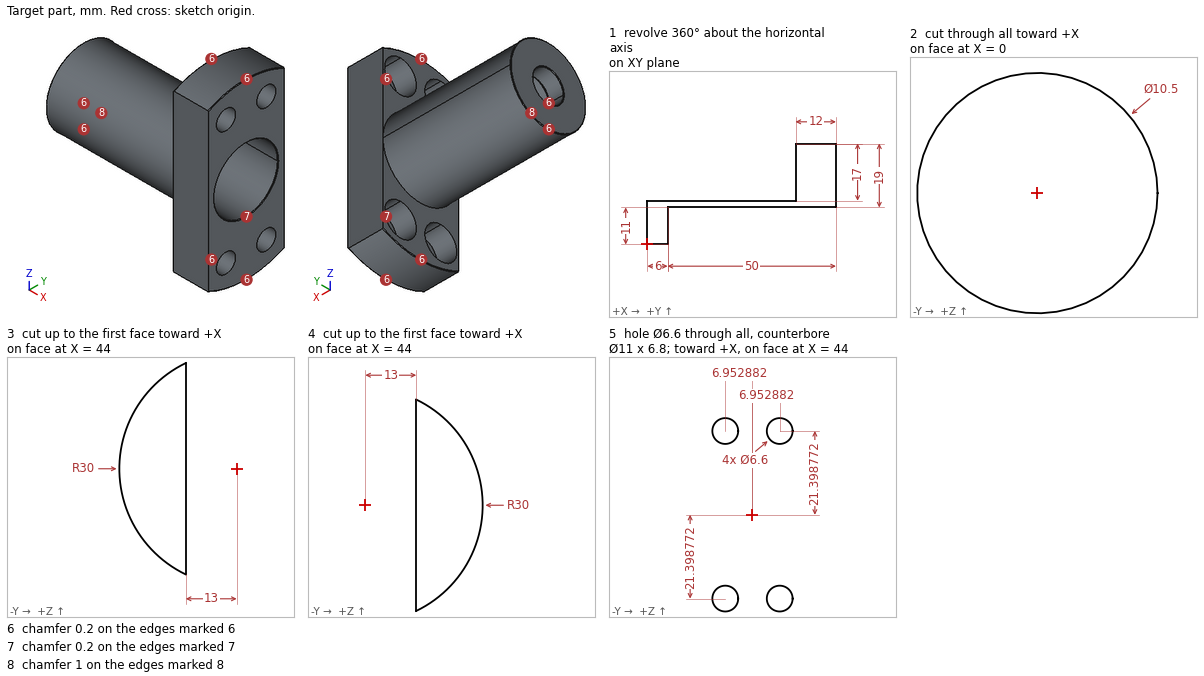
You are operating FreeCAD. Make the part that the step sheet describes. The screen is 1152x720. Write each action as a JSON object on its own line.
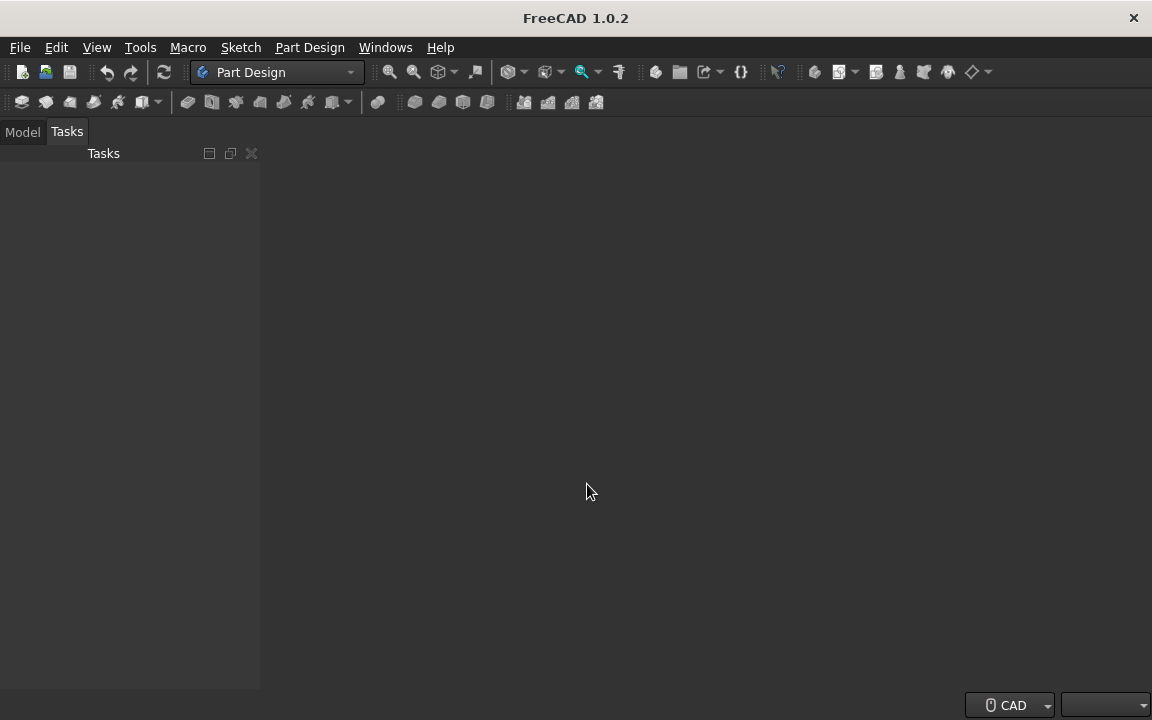
{"action": "left_click", "coordinate": [22, 72]}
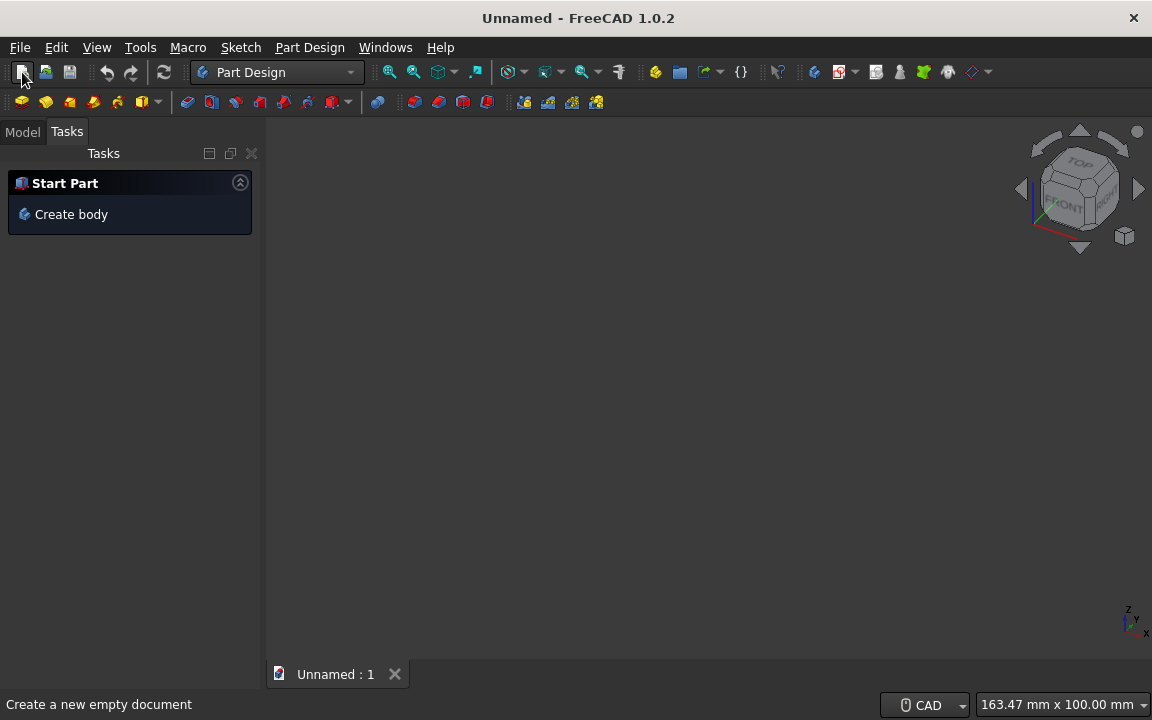
{"action": "left_click", "coordinate": [840, 72]}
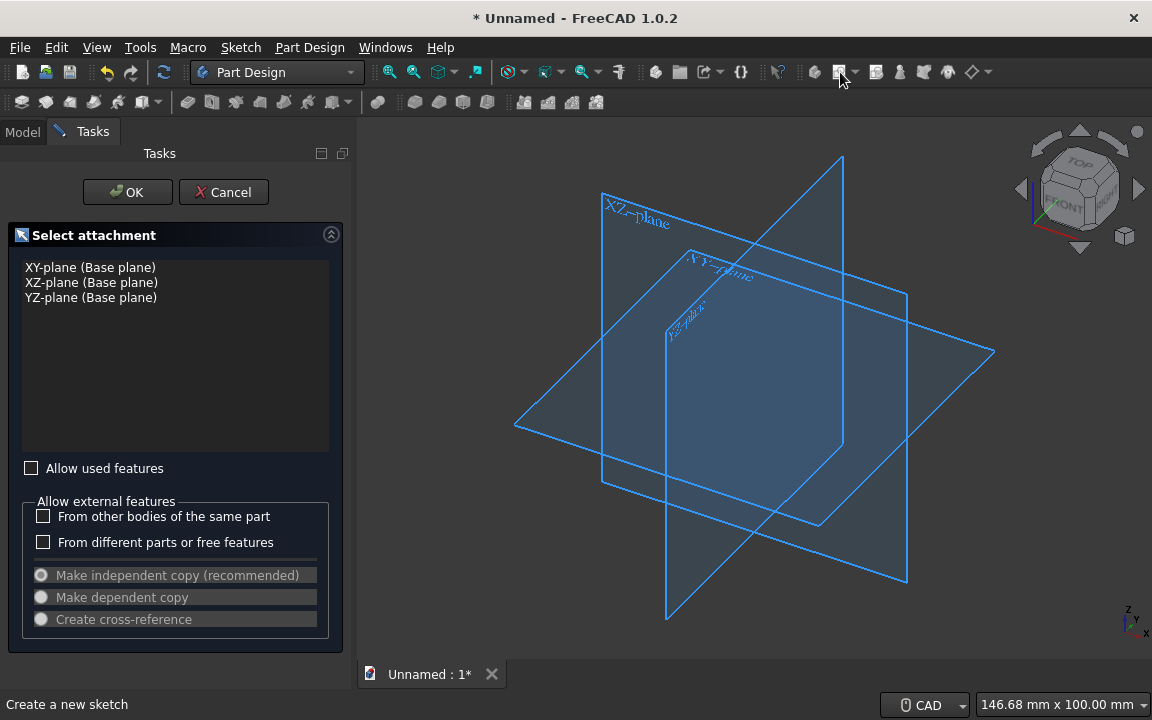
{"action": "left_click", "coordinate": [82, 268]}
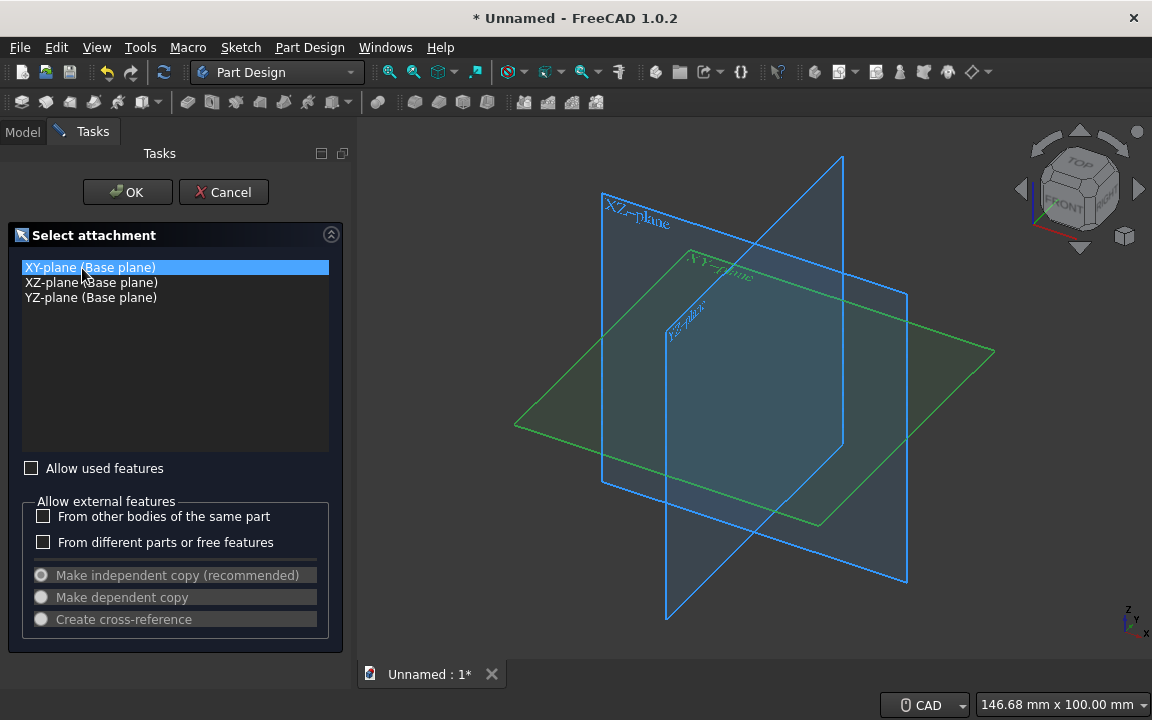
{"action": "left_click", "coordinate": [128, 192]}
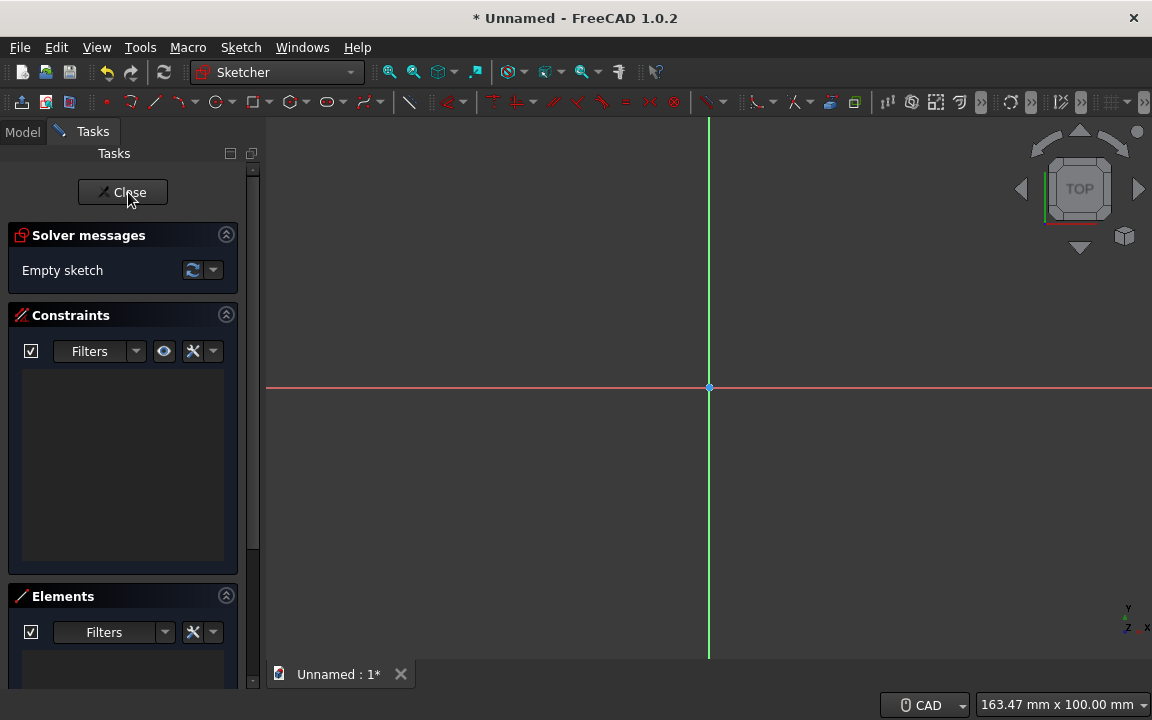
{"action": "scroll", "coordinate": [294, 631], "scroll_direction": "down", "scroll_amount": 1}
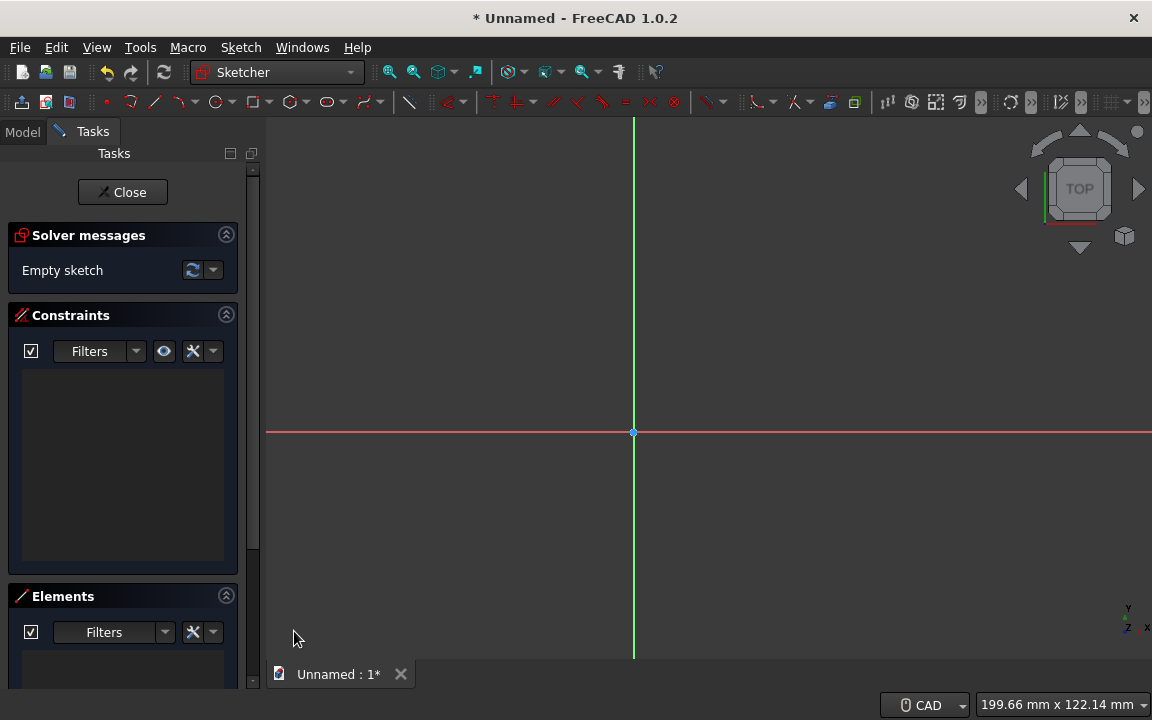
{"action": "scroll", "coordinate": [901, 338], "scroll_direction": "up", "scroll_amount": 3}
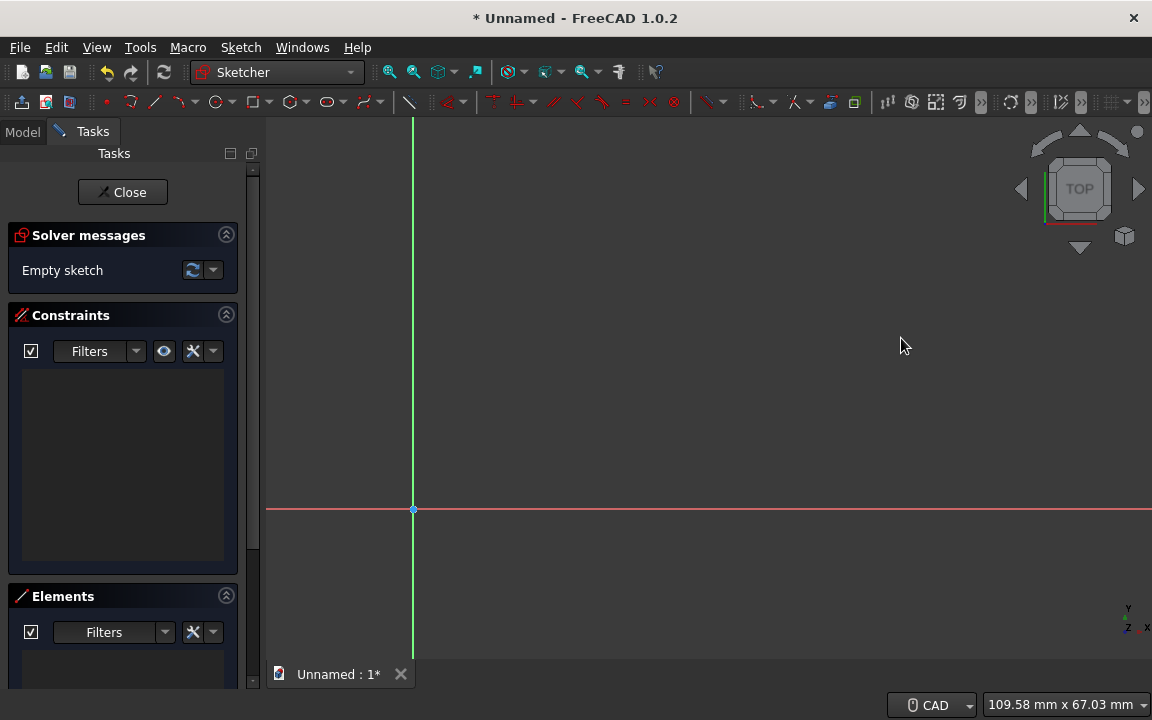
{"action": "left_click", "coordinate": [132, 102]}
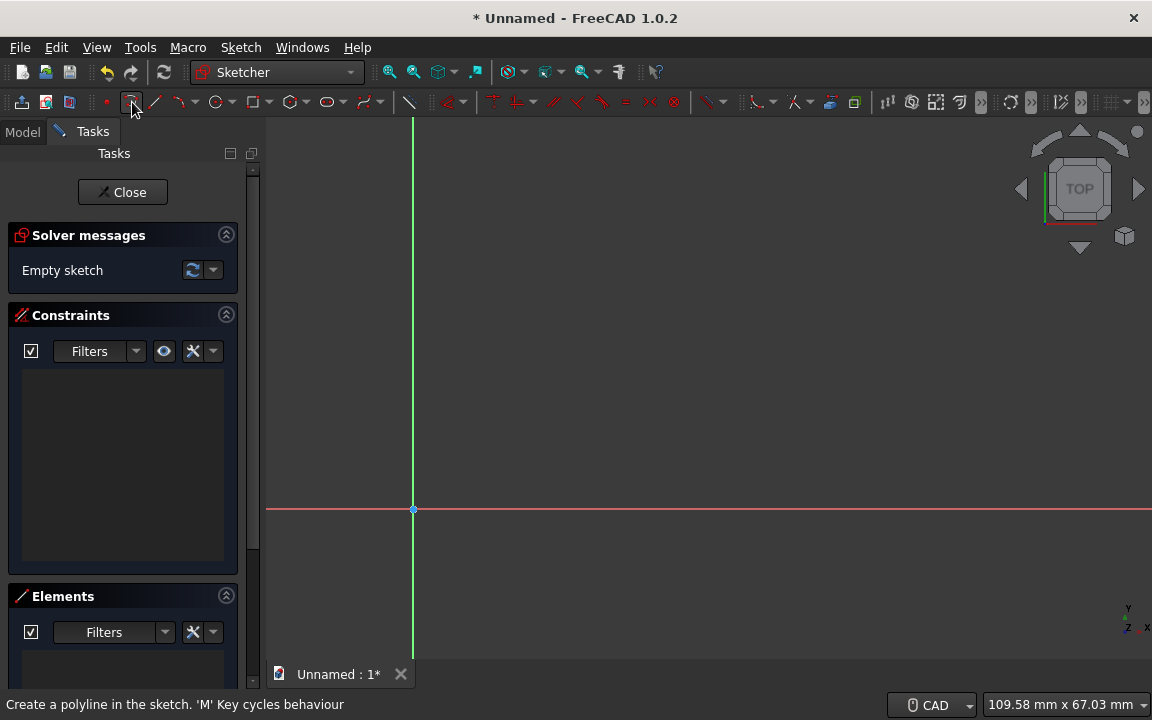
{"action": "left_click", "coordinate": [414, 509]}
{"action": "left_click", "coordinate": [462, 500]}
{"action": "left_click", "coordinate": [462, 420]}
{"action": "left_click", "coordinate": [866, 420]}
{"action": "left_click", "coordinate": [866, 267]}
{"action": "left_click", "coordinate": [769, 267]}
{"action": "left_click", "coordinate": [769, 404]}
{"action": "left_click", "coordinate": [423, 404]}
{"action": "left_click", "coordinate": [414, 509]}
{"action": "key", "text": "Escape"}
{"action": "key", "text": "Escape"}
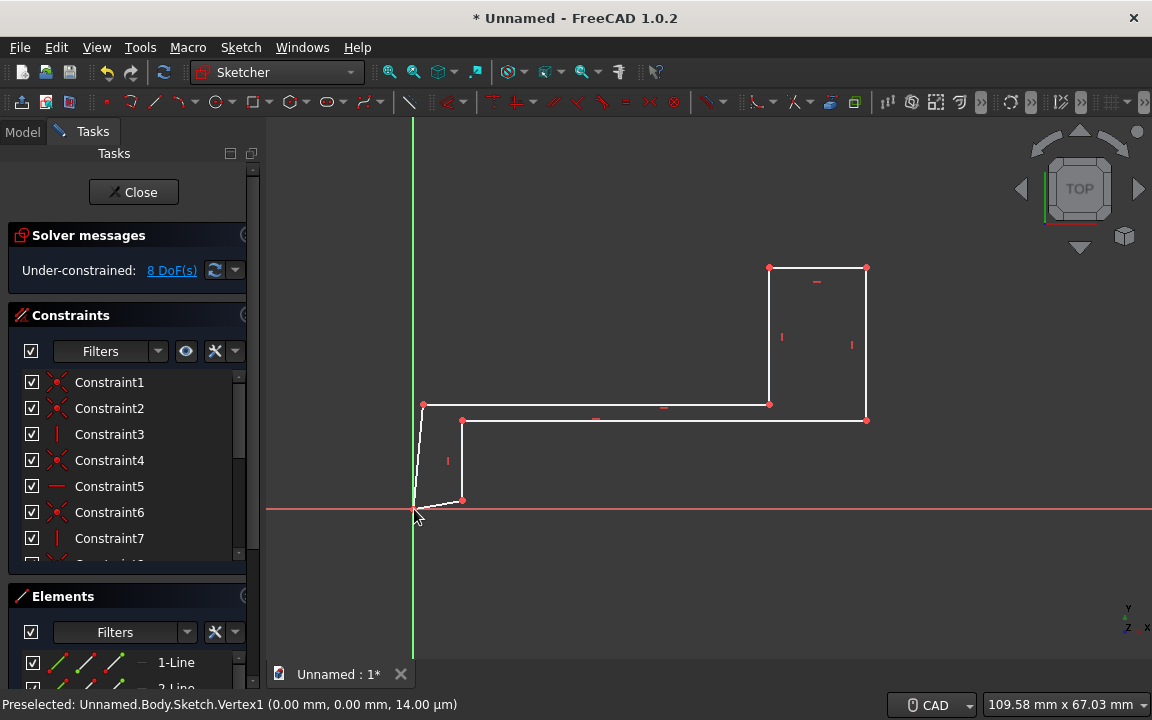
{"action": "left_click", "coordinate": [428, 507]}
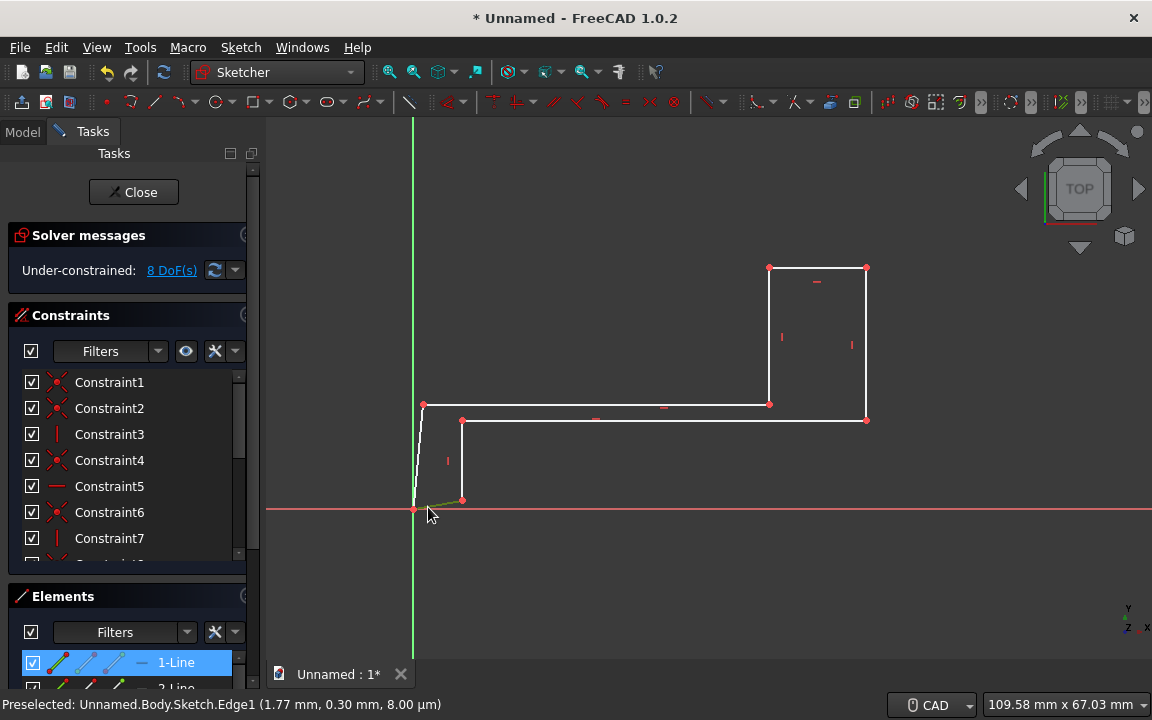
{"action": "key", "text": "h"}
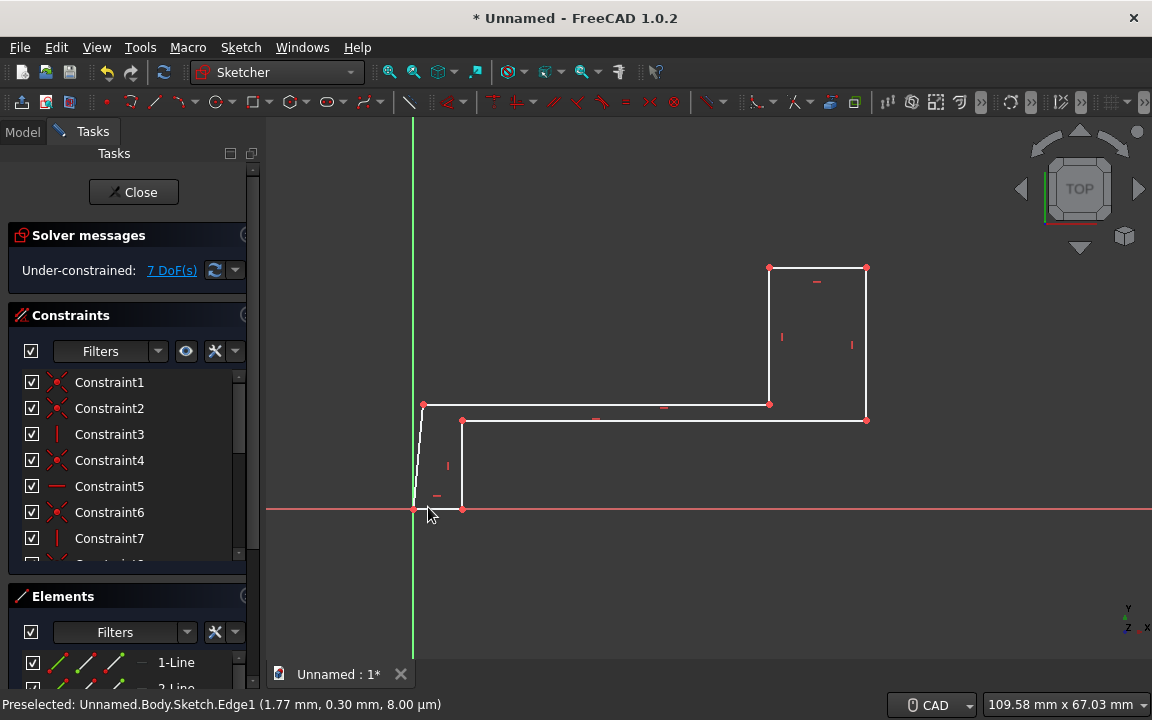
{"action": "left_click", "coordinate": [416, 478]}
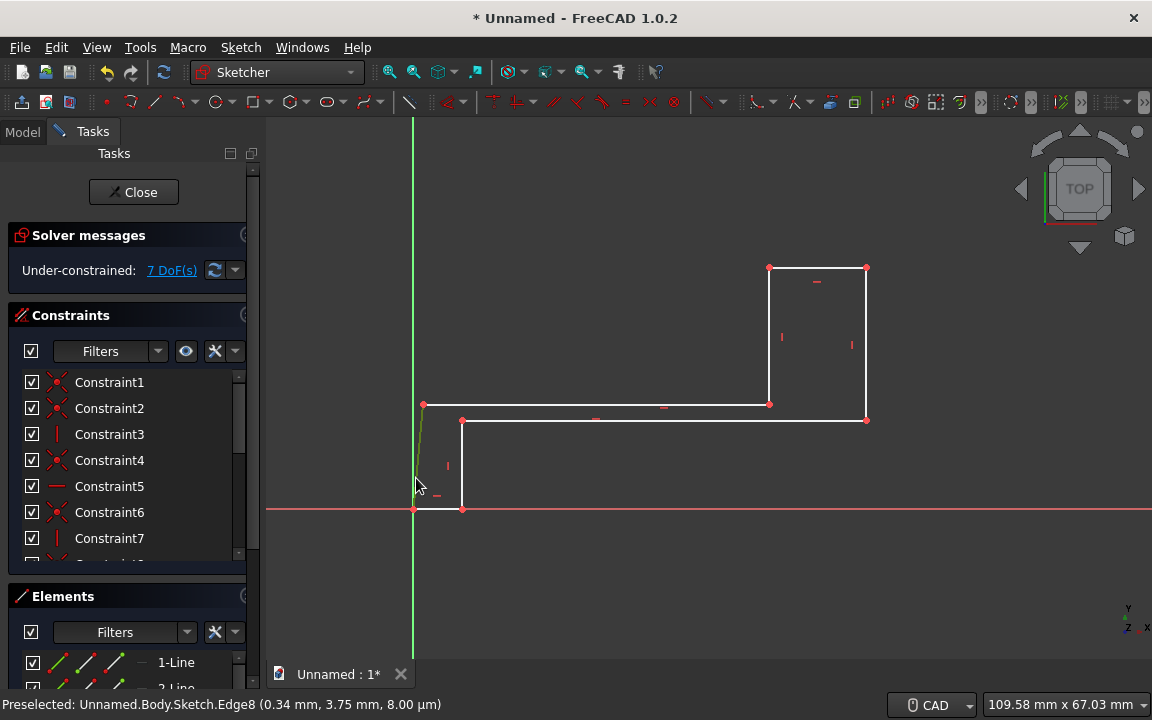
{"action": "left_click", "coordinate": [536, 102]}